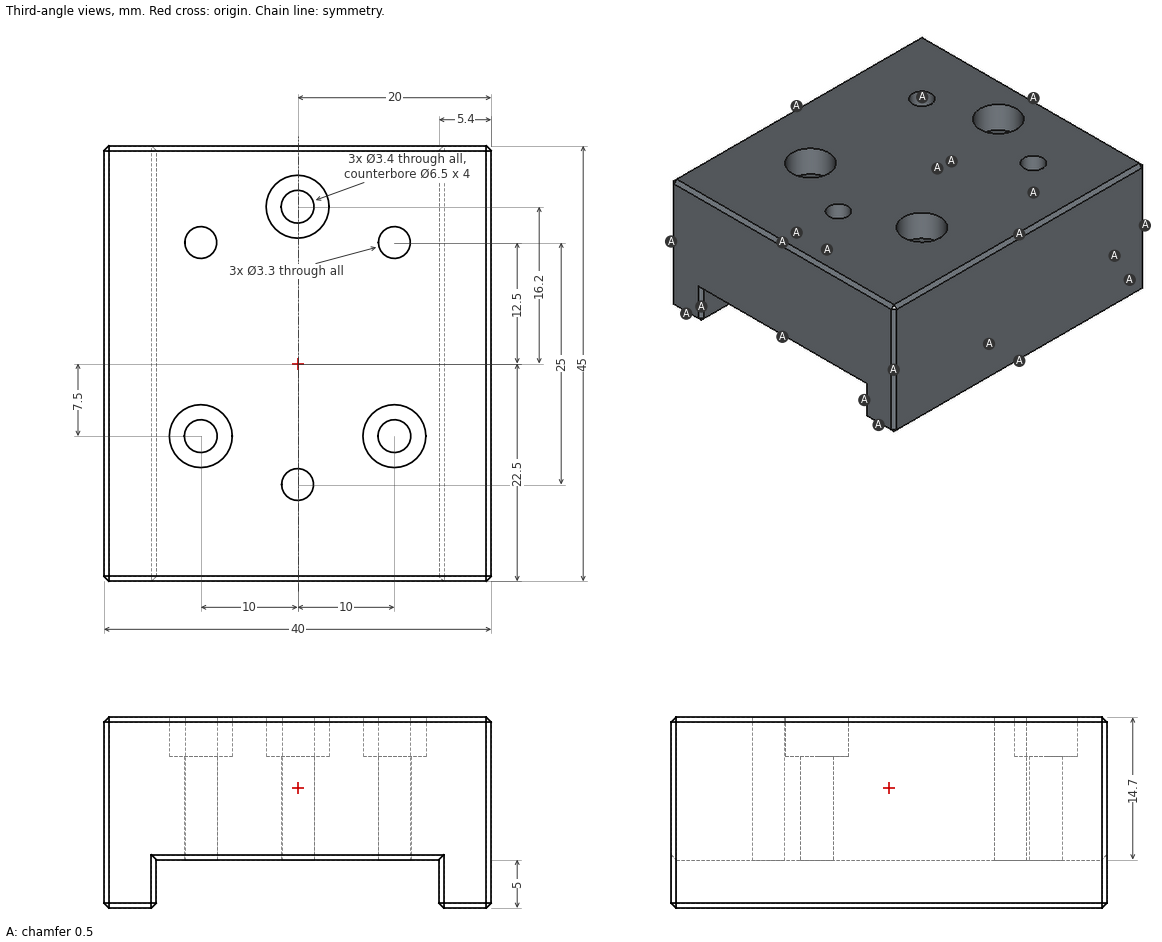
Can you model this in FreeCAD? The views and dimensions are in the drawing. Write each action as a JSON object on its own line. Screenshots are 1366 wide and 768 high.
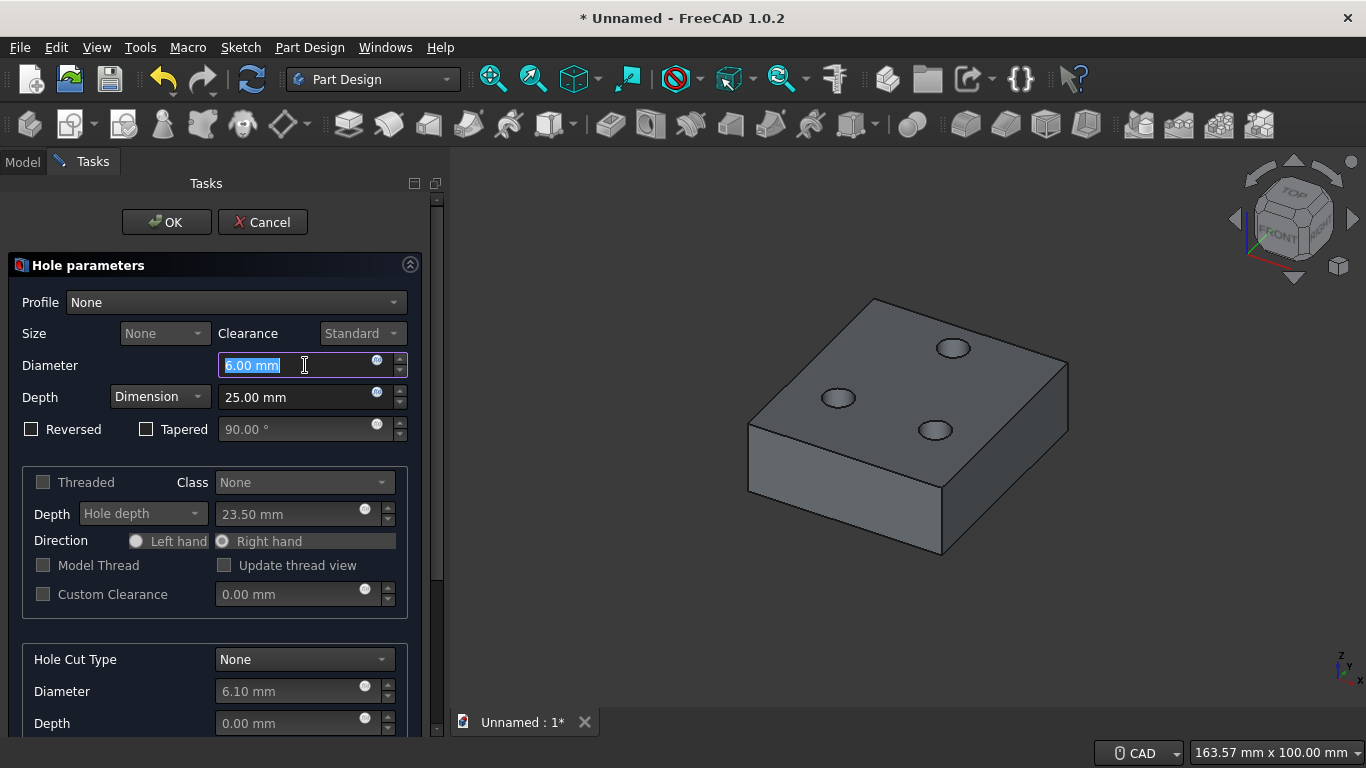
{"action": "type", "text": "3.4"}
{"action": "key", "text": "Tab"}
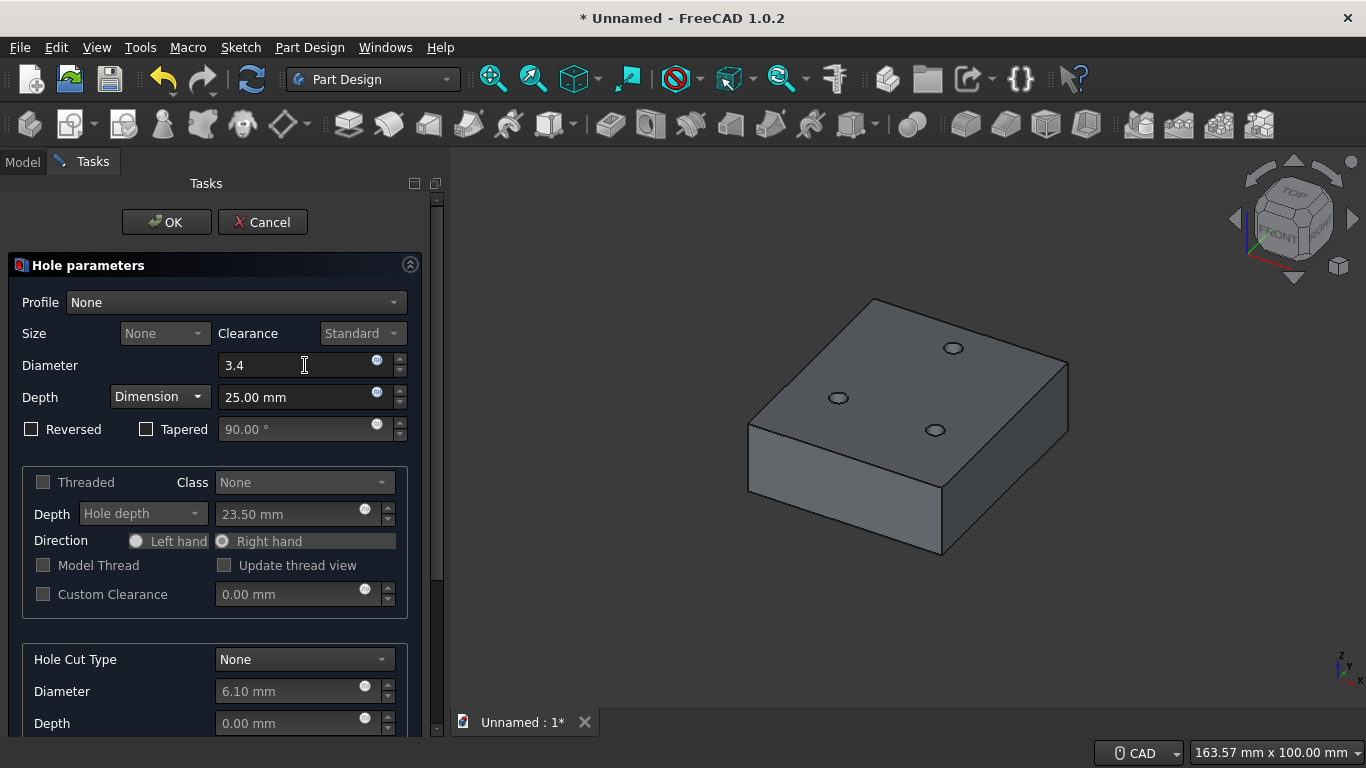
{"action": "left_click", "coordinate": [161, 396]}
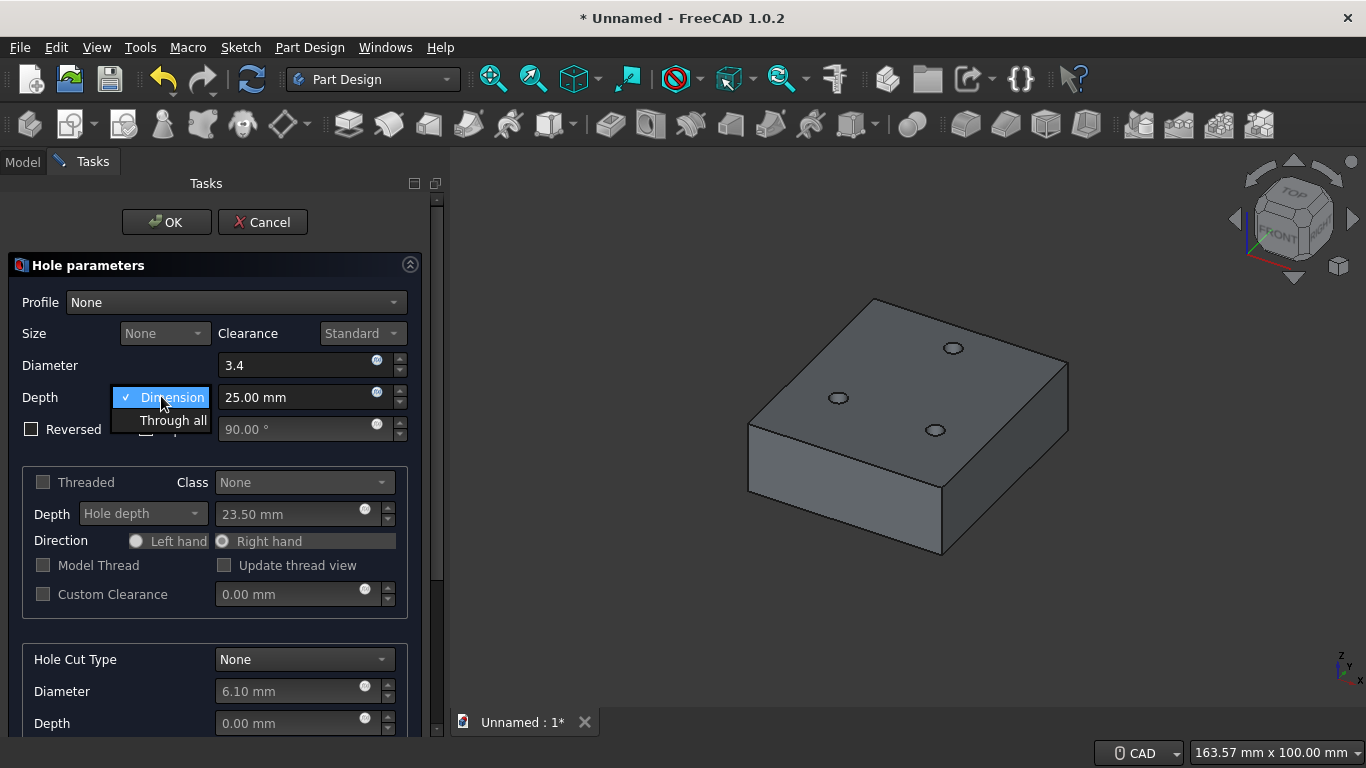
{"action": "left_click", "coordinate": [160, 420]}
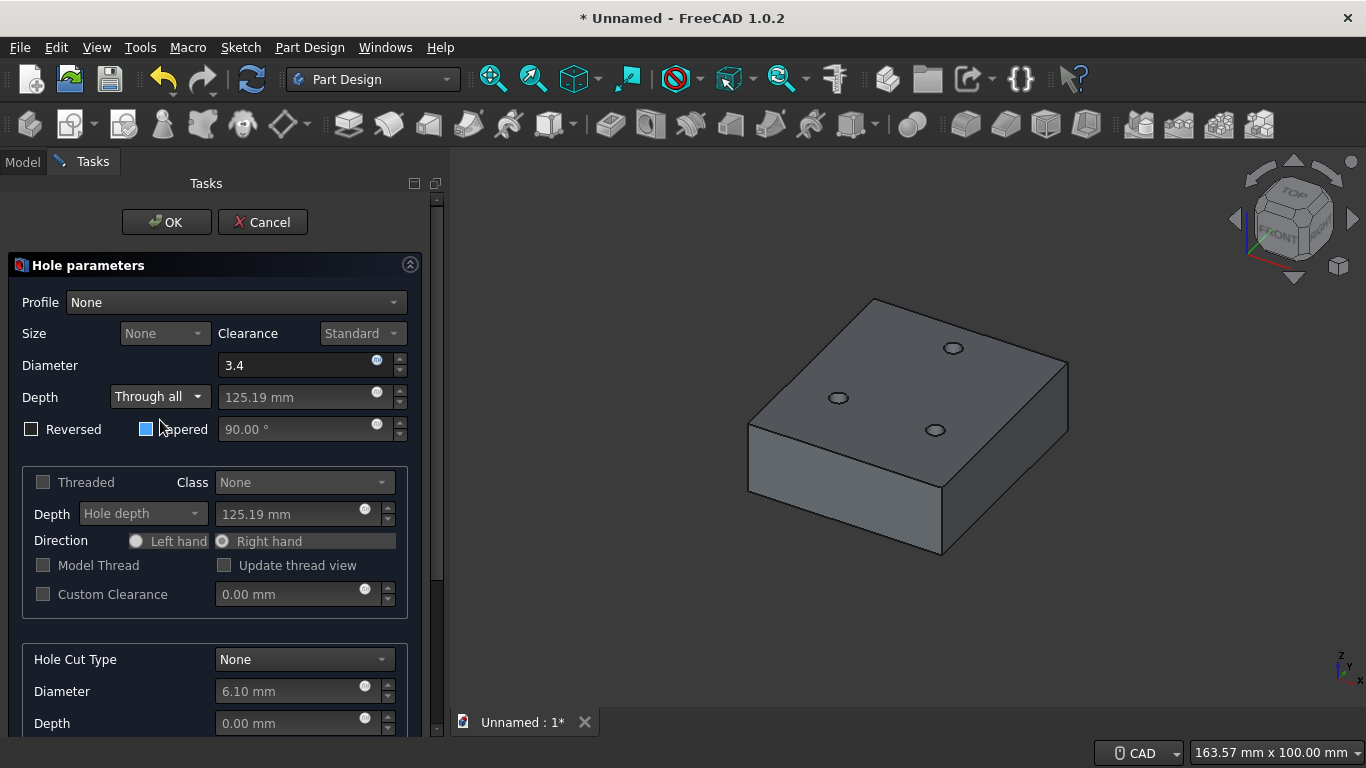
{"action": "left_click", "coordinate": [306, 660]}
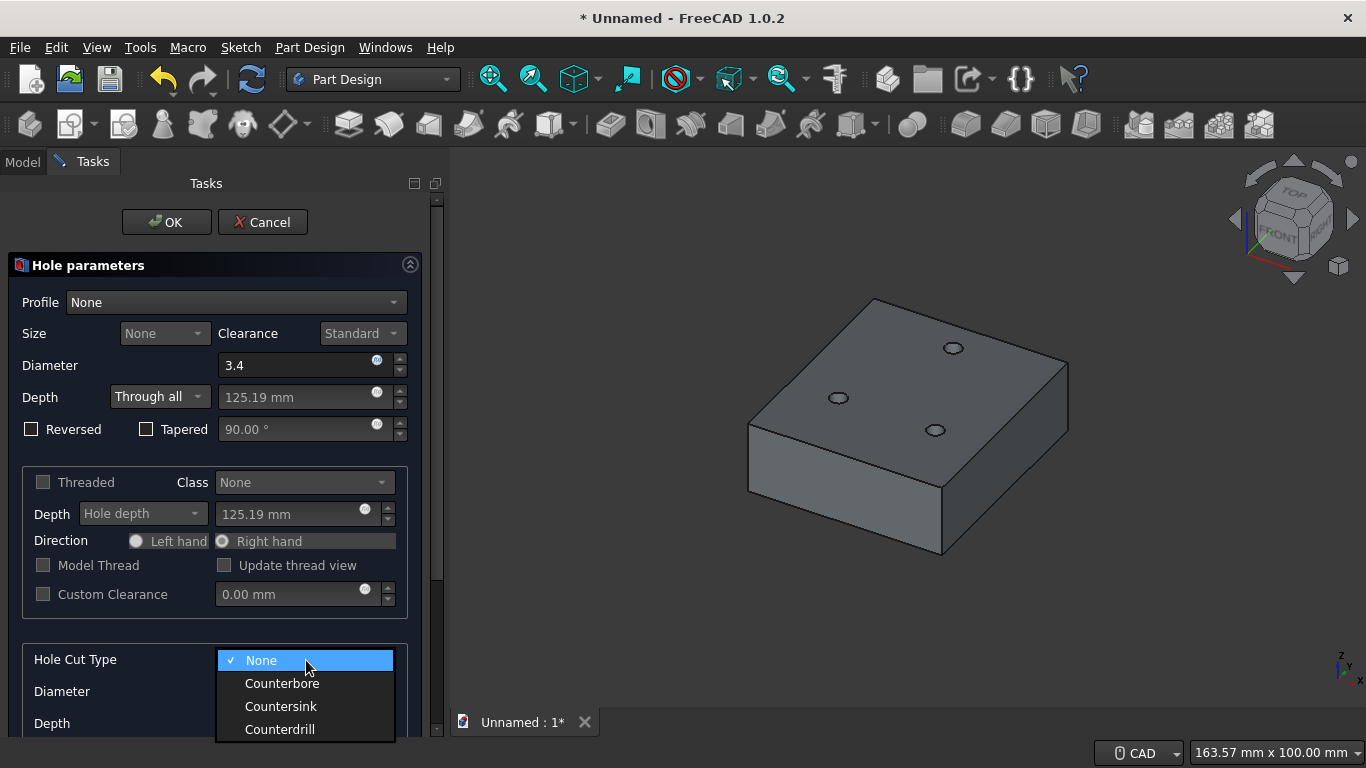
{"action": "left_click", "coordinate": [304, 684]}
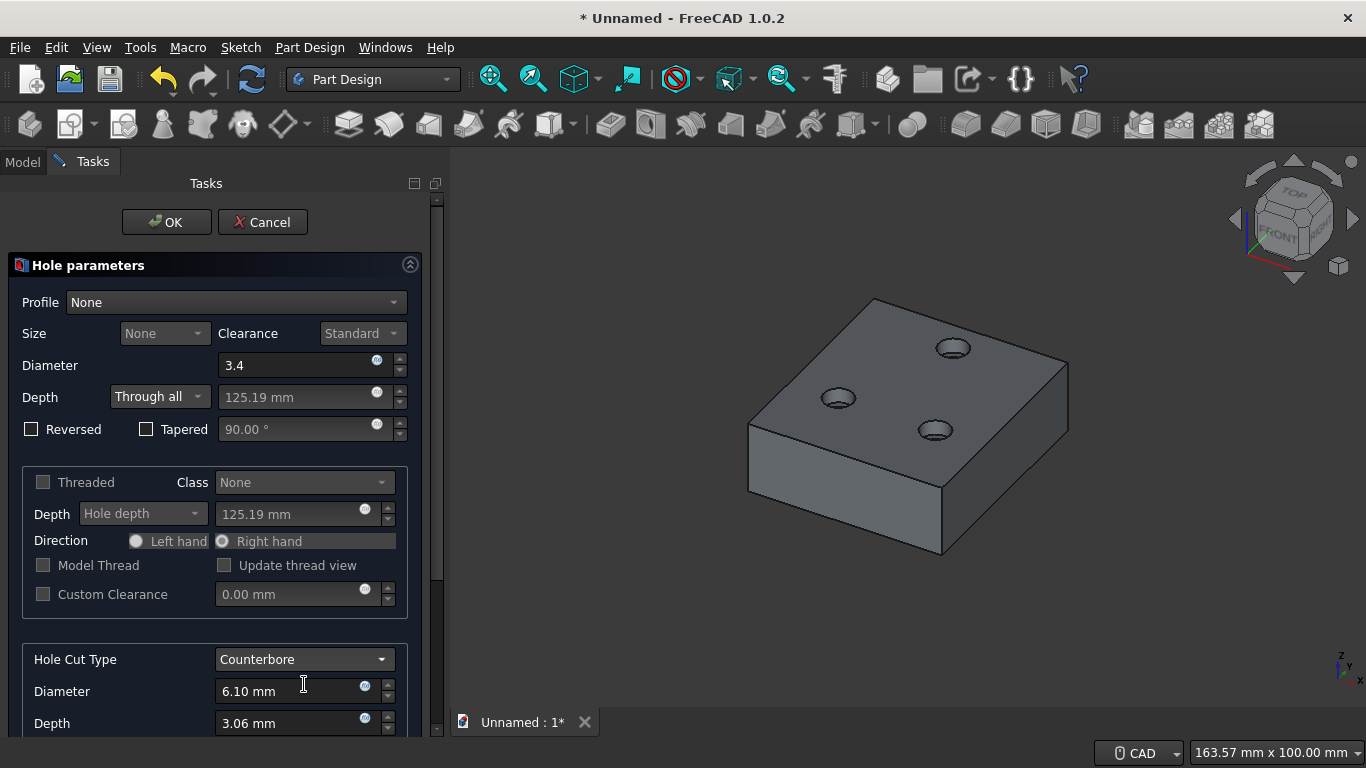
{"action": "triple_click", "coordinate": [298, 691]}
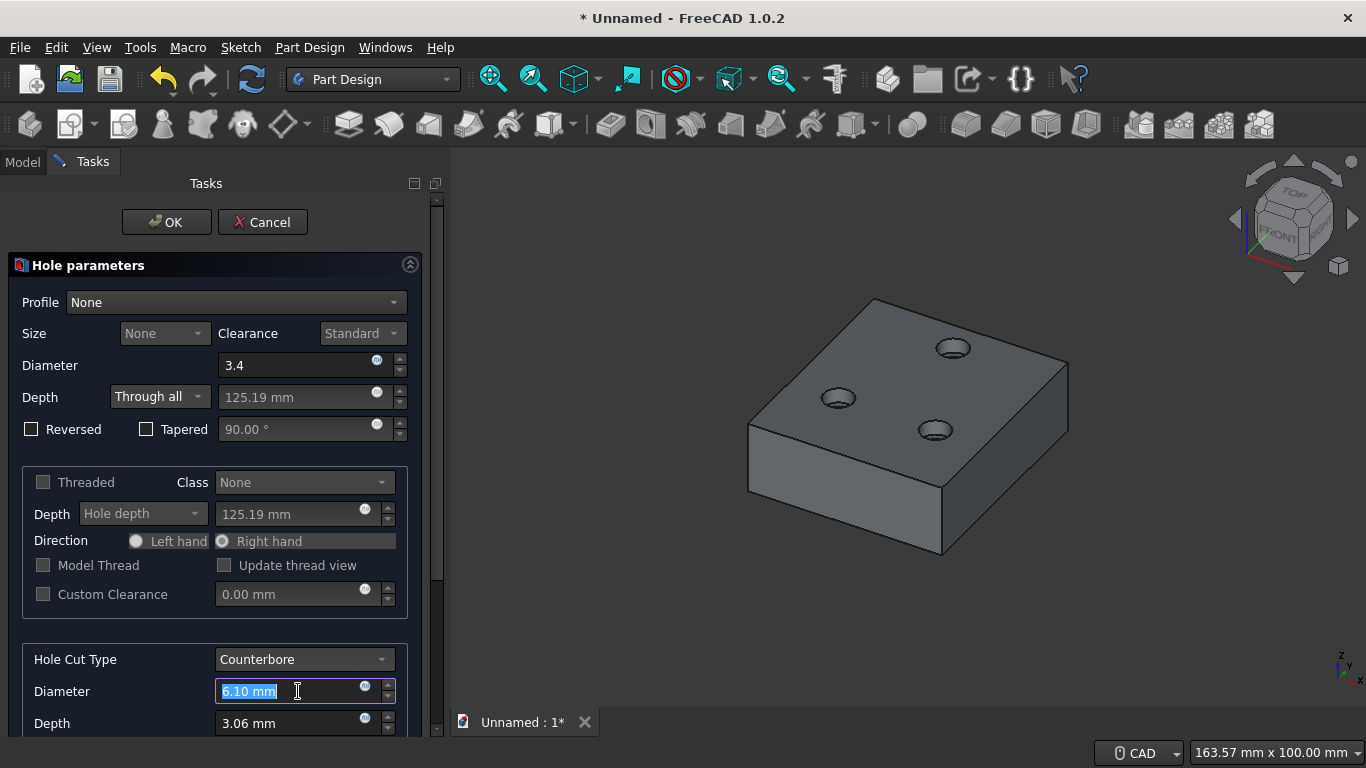
{"action": "type", "text": "6.5"}
{"action": "key", "text": "Tab"}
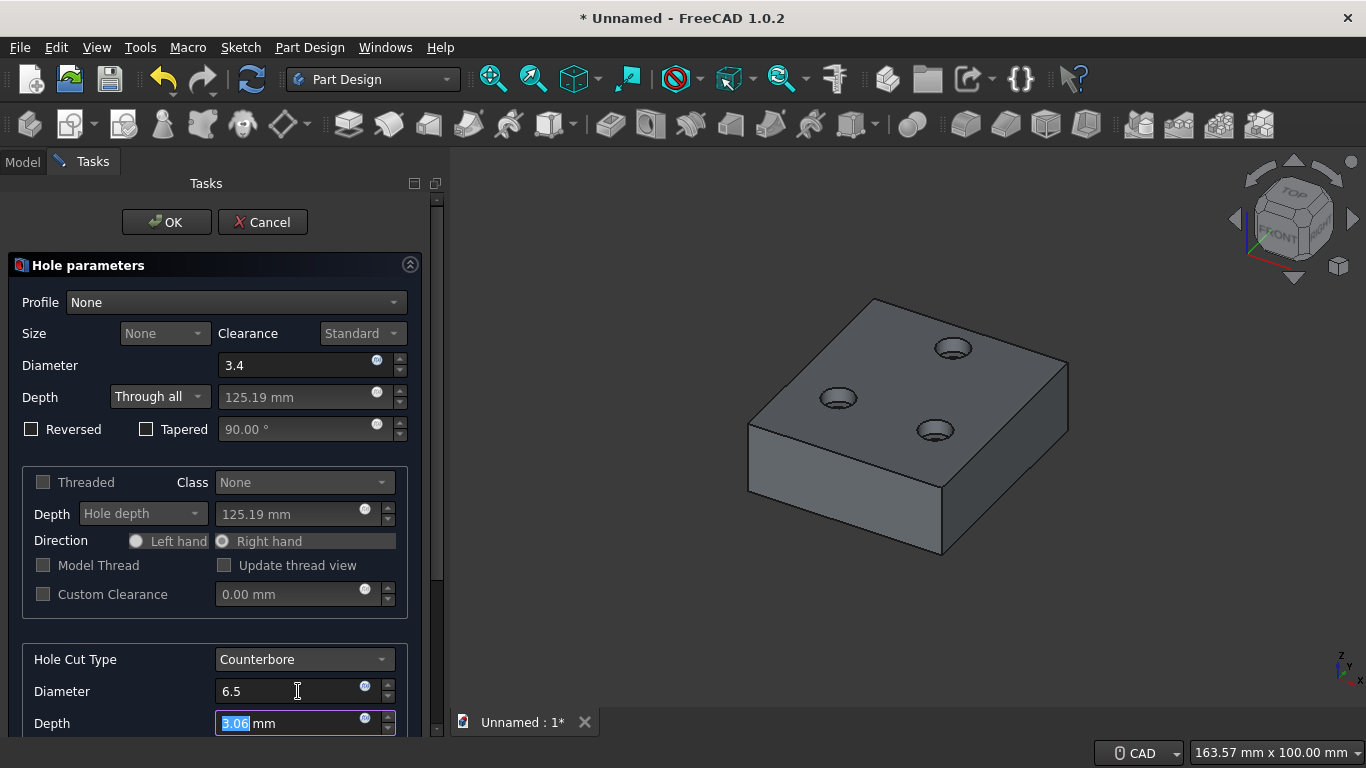
{"action": "type", "text": "4"}
{"action": "key", "text": "Tab"}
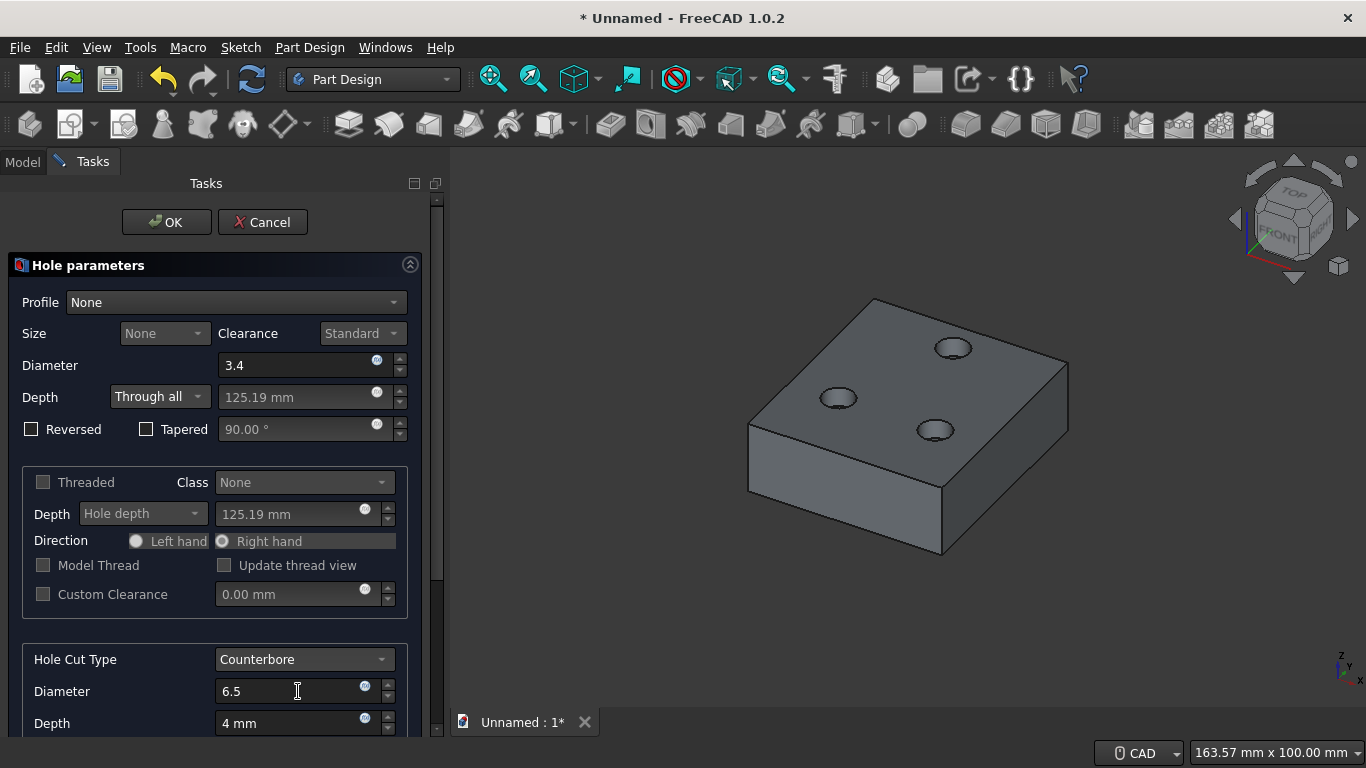
{"action": "left_click", "coordinate": [167, 222]}